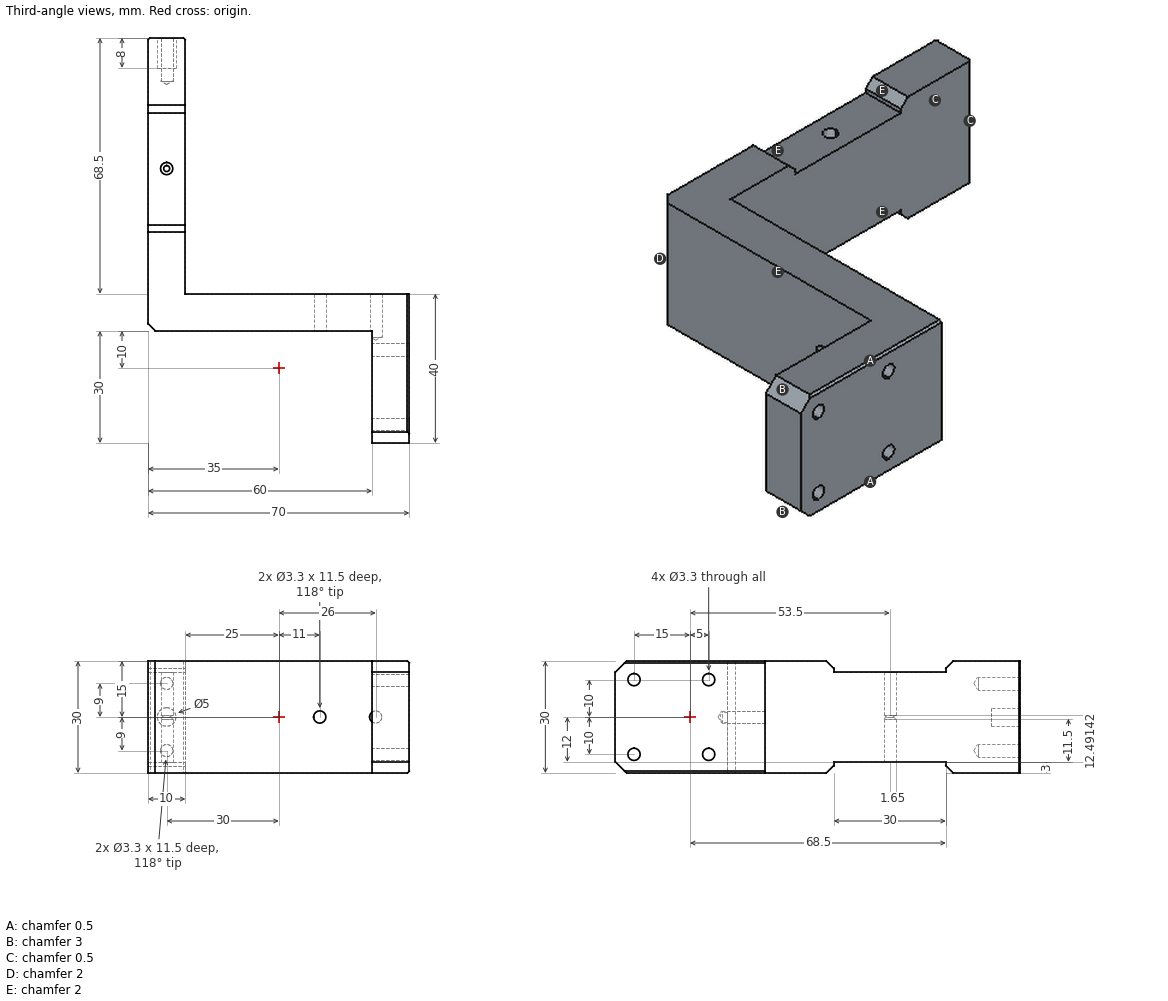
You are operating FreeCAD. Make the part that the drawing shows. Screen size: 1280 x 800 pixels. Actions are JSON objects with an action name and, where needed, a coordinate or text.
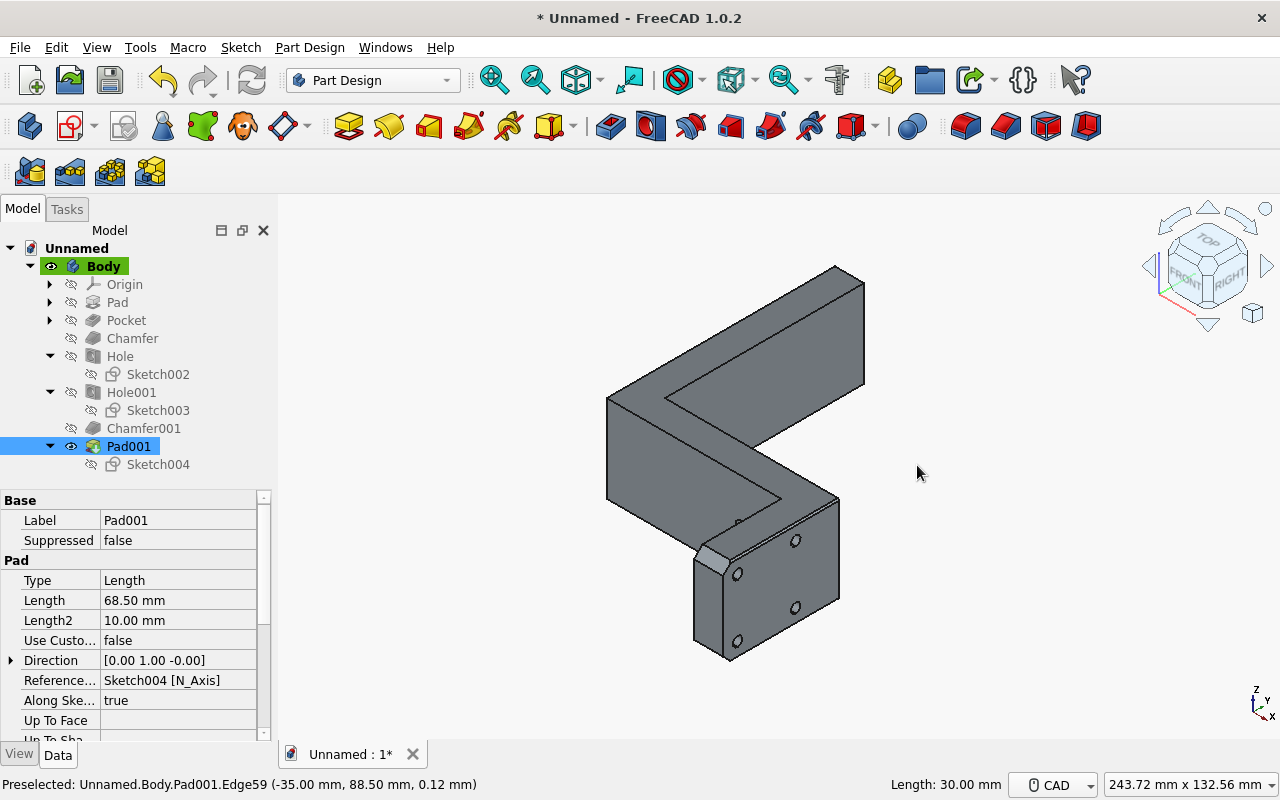
{"action": "key", "text": "2"}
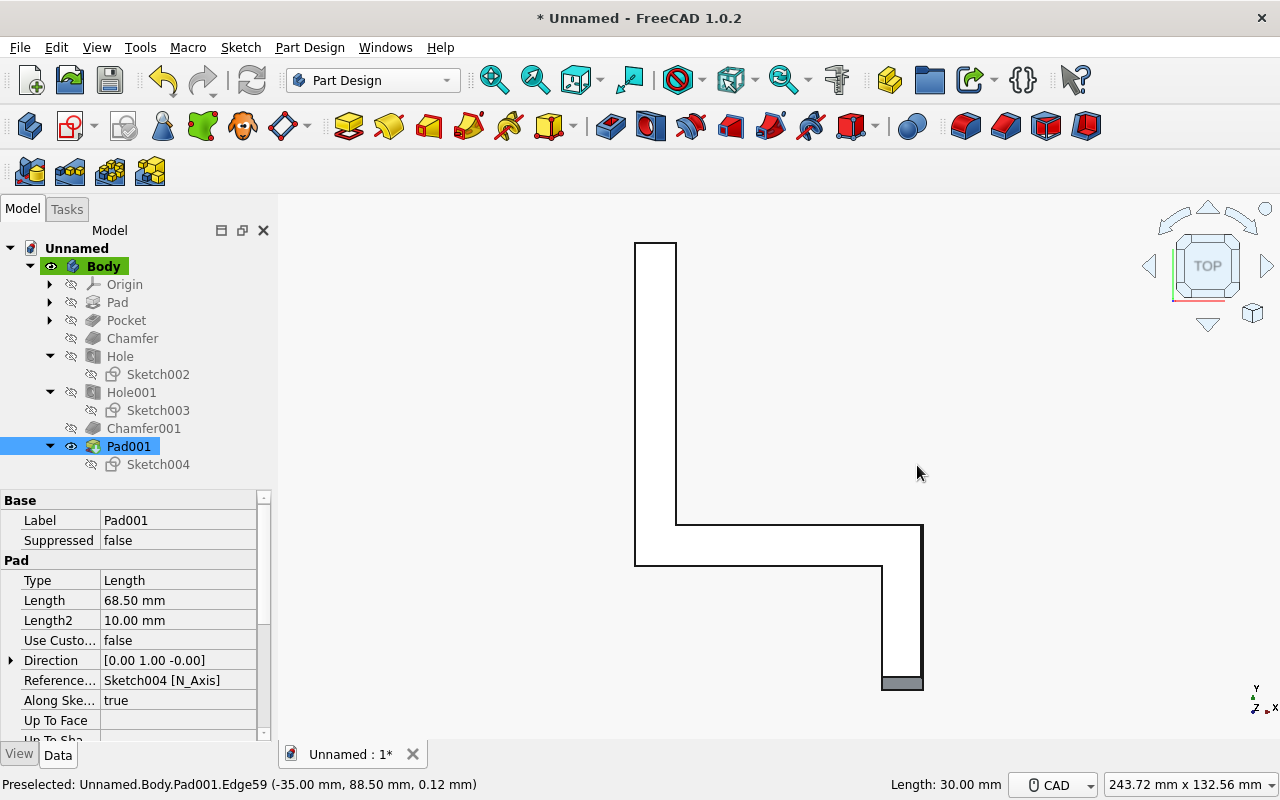
{"action": "key", "text": "1"}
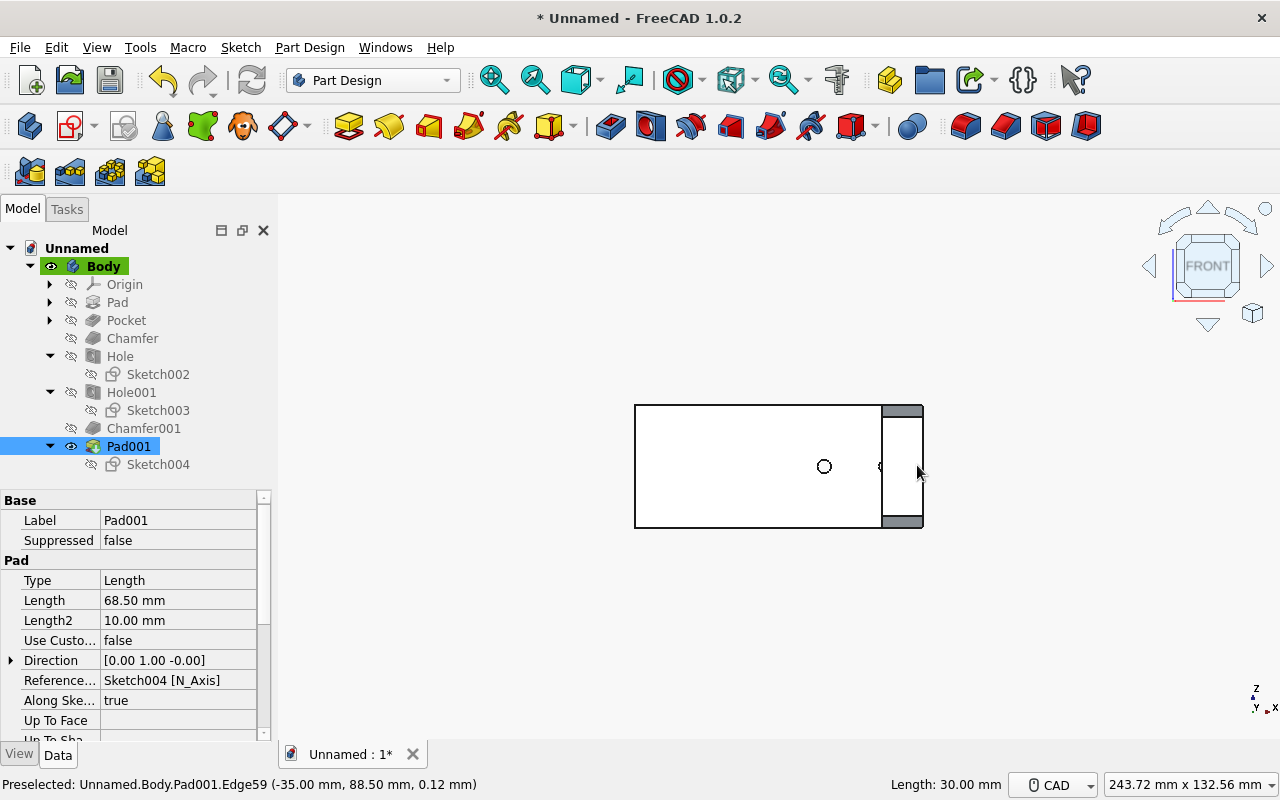
{"action": "left_click", "coordinate": [496, 80]}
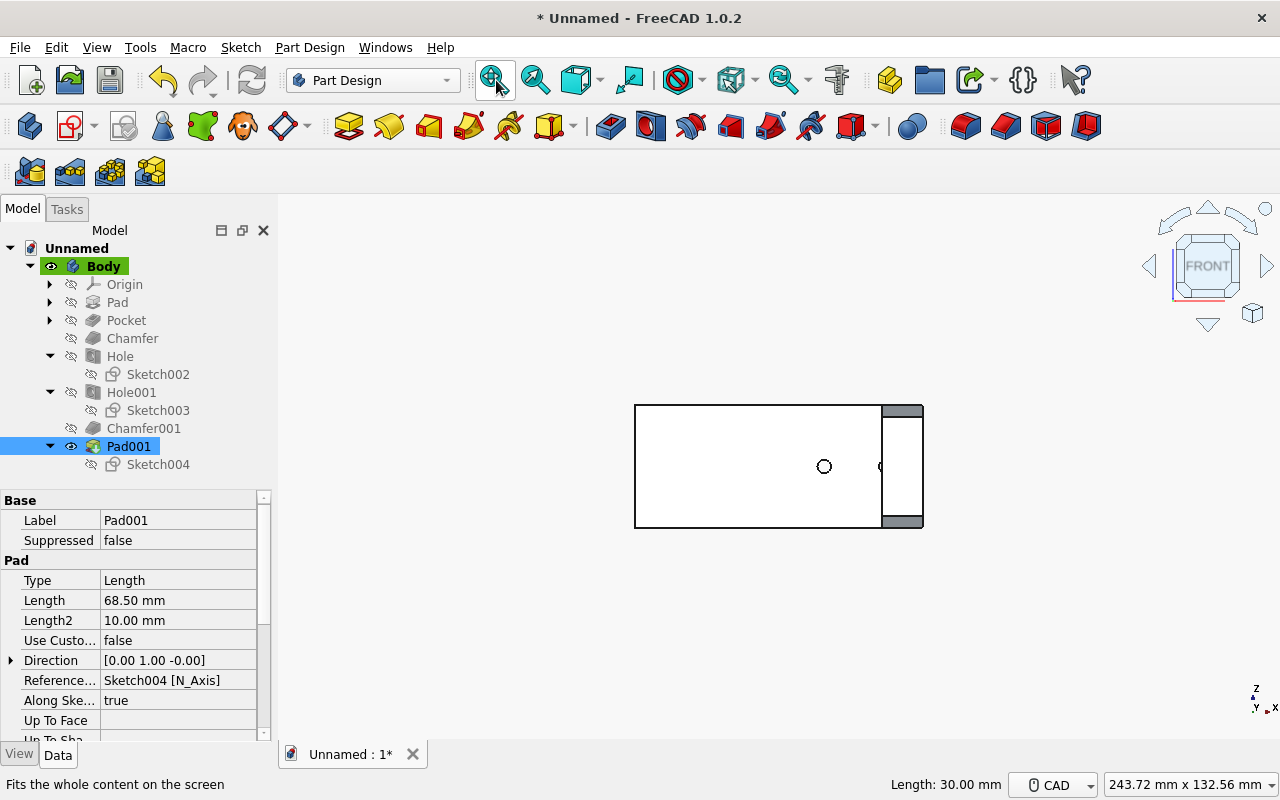
{"action": "key", "text": "3"}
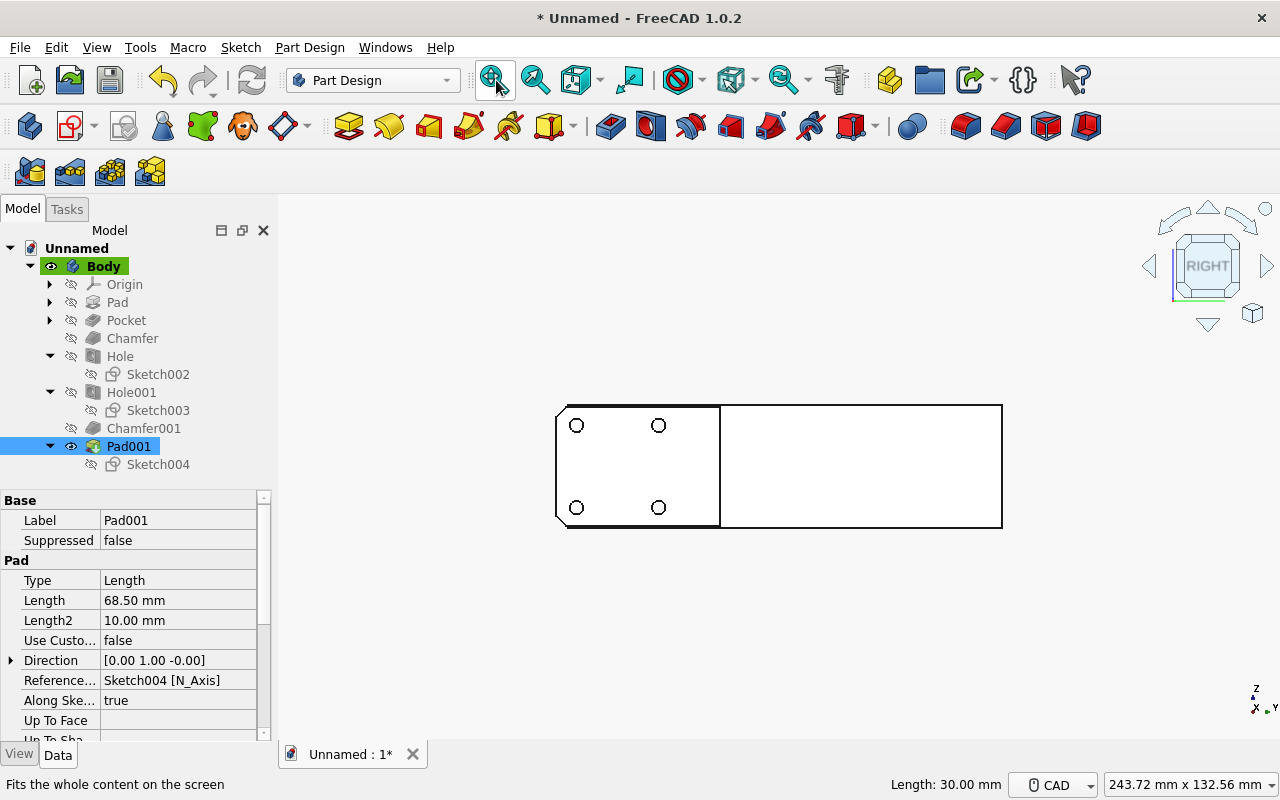
{"action": "key", "text": "v f"}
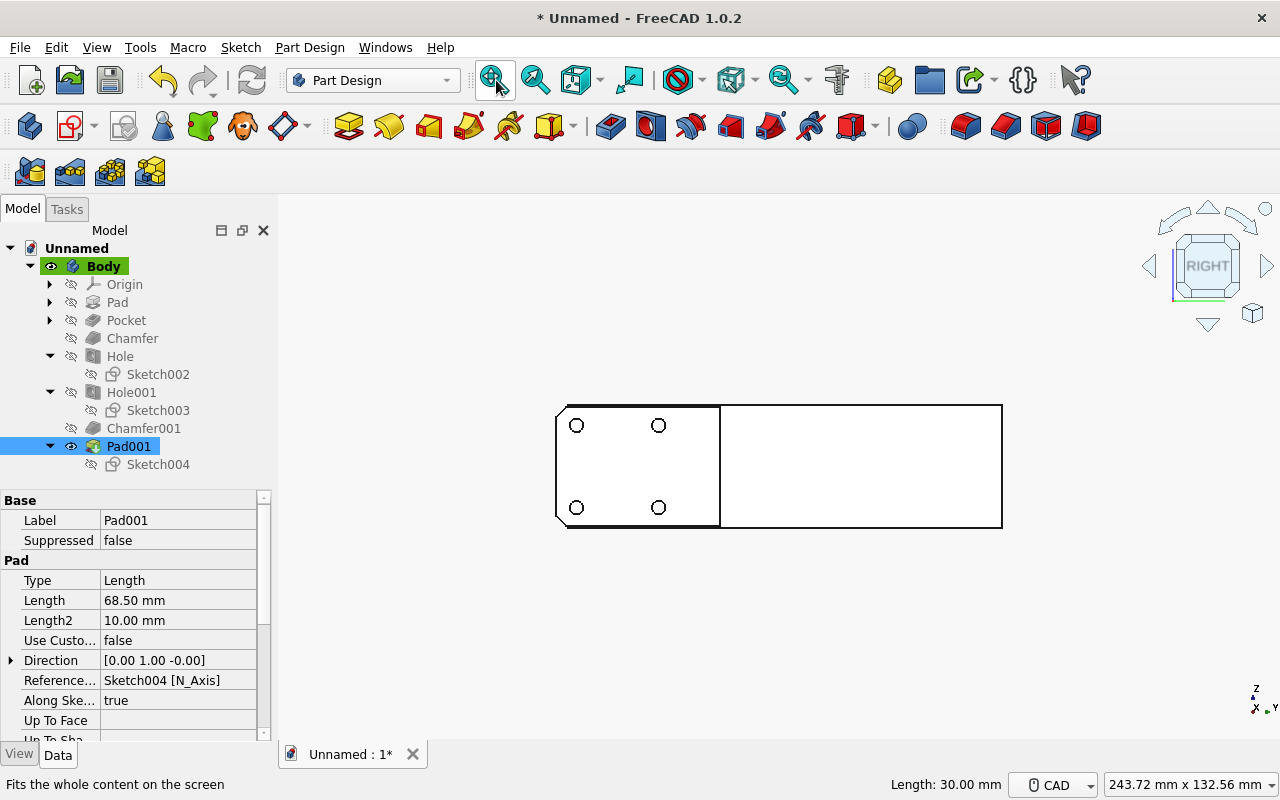
{"action": "left_click", "coordinate": [1002, 465], "text": "ctrl"}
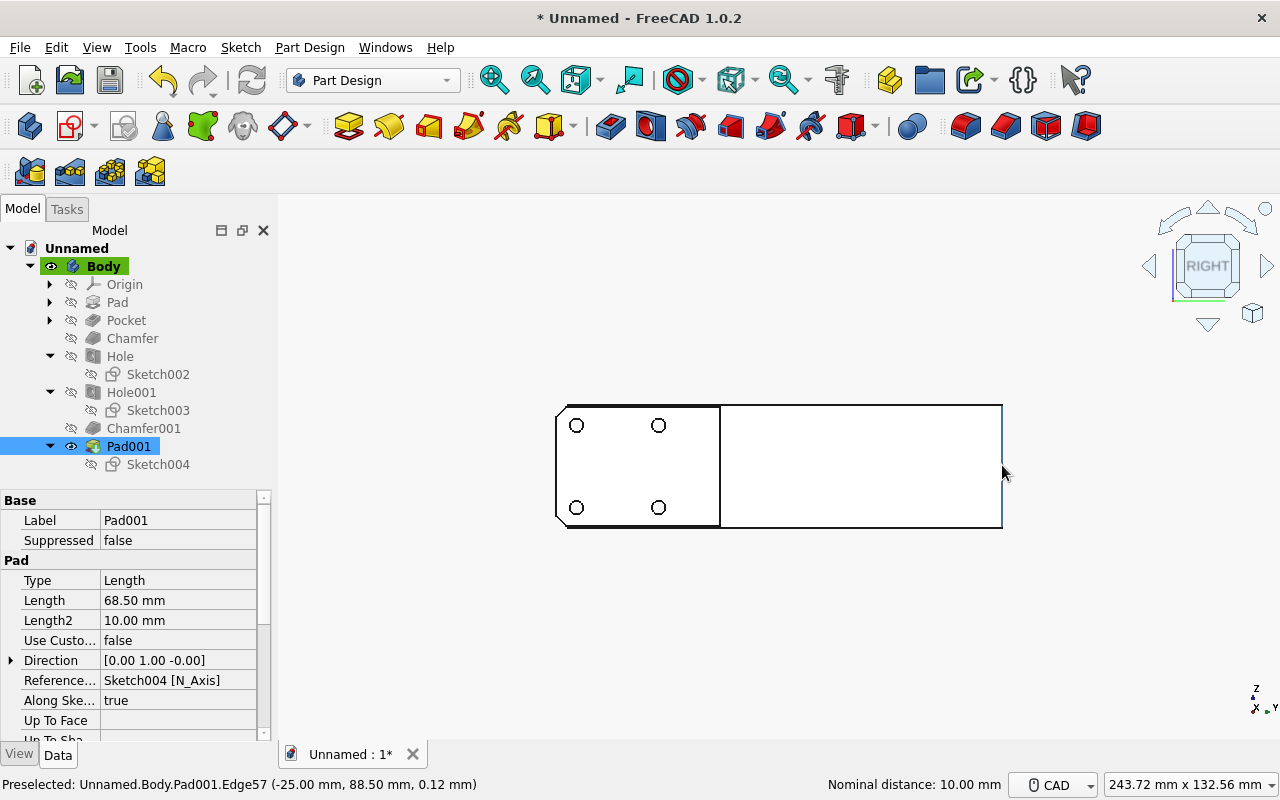
{"action": "left_click", "coordinate": [1006, 126]}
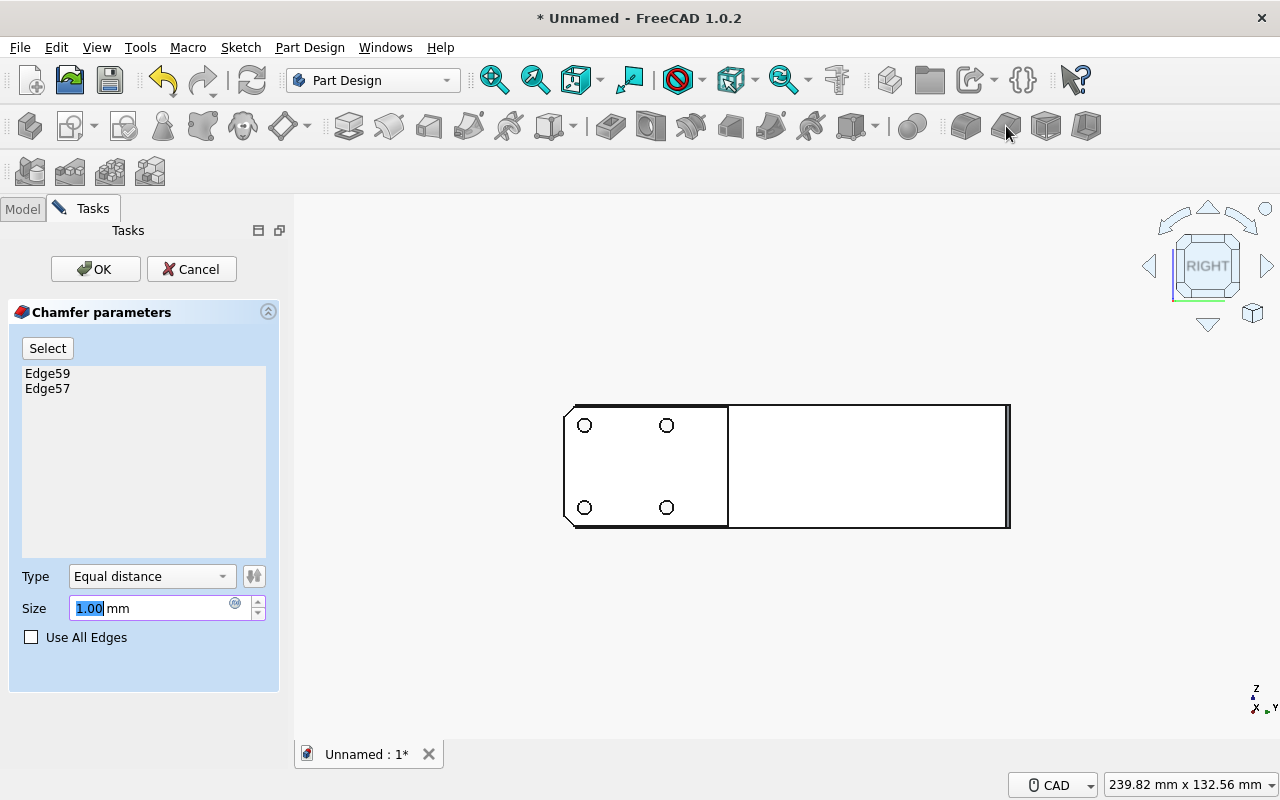
{"action": "type", "text": "0.5"}
{"action": "key", "text": "Tab"}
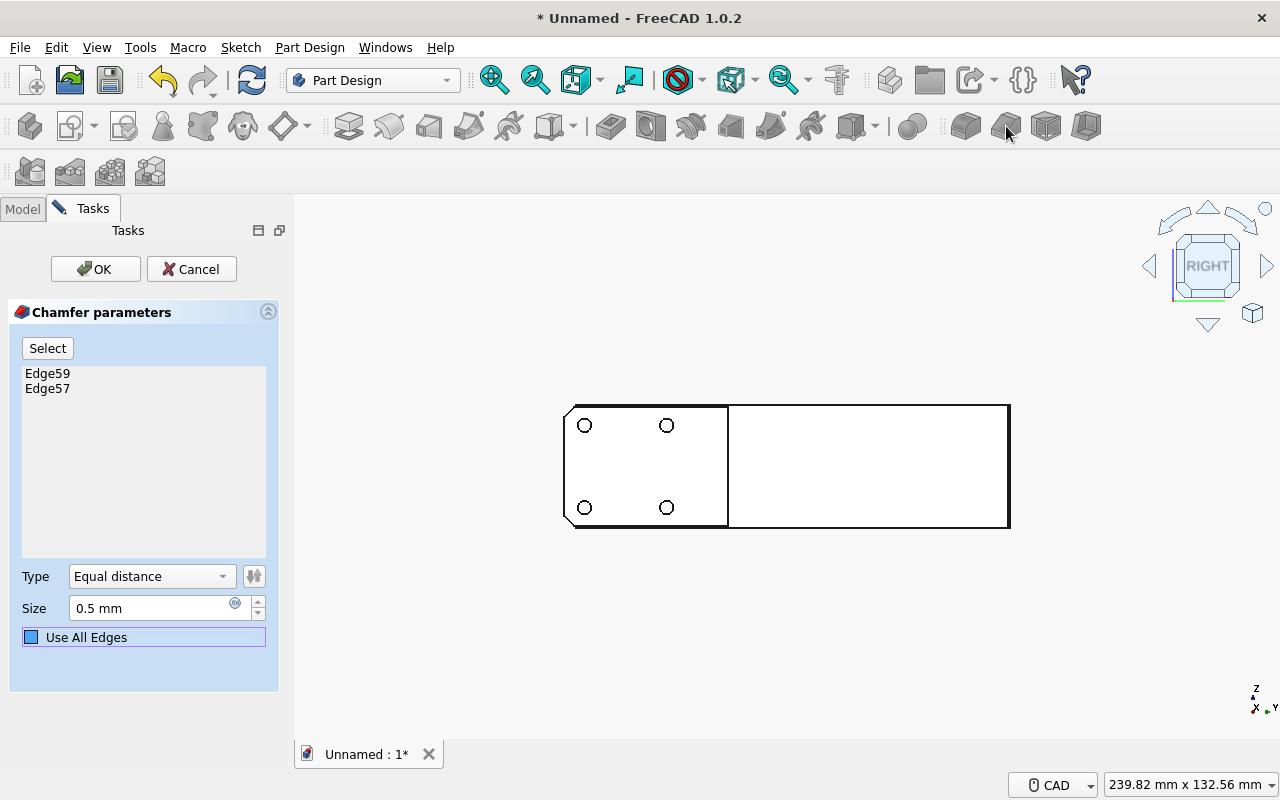
{"action": "left_click", "coordinate": [96, 269]}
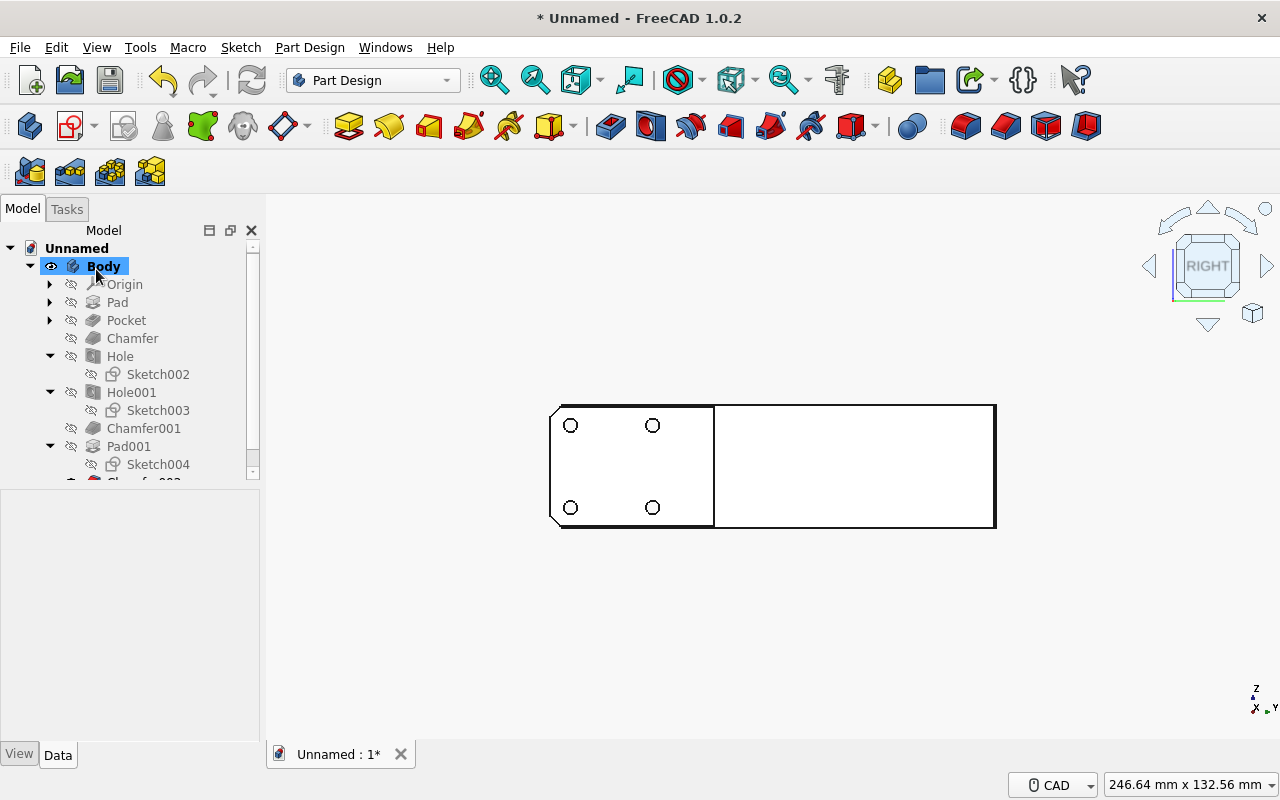
{"action": "left_click", "coordinate": [496, 80]}